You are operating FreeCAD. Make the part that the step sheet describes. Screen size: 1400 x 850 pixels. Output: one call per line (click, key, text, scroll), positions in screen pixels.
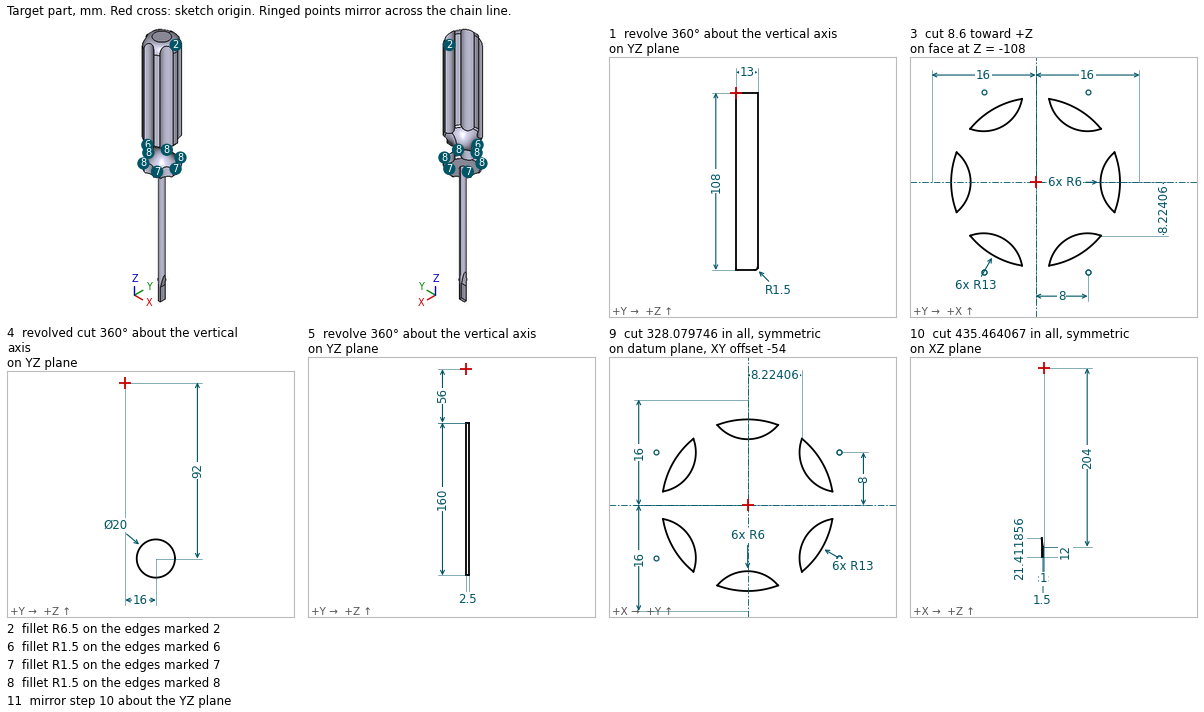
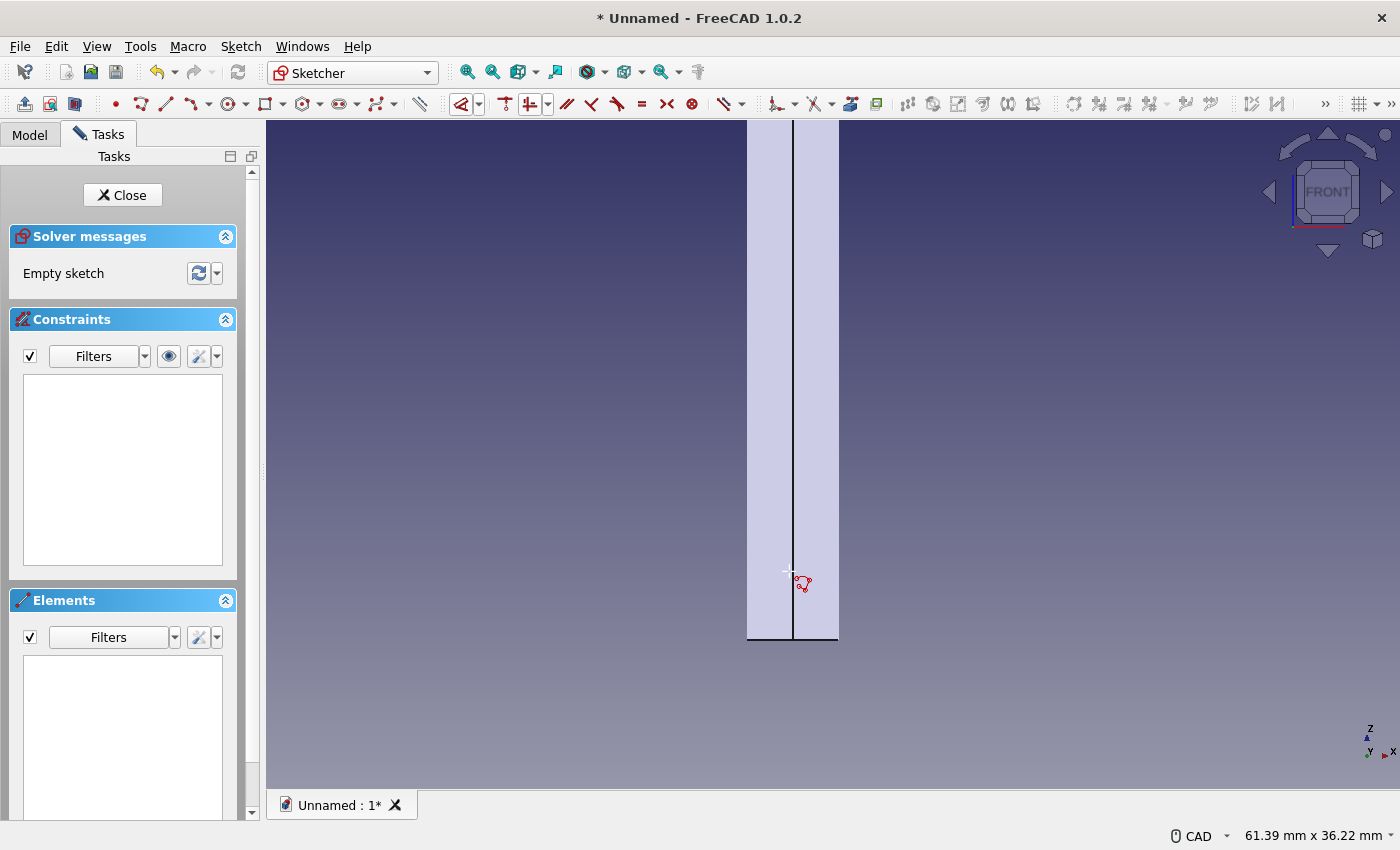
click(747, 244)
click(774, 418)
click(774, 640)
click(747, 640)
click(747, 245)
key(Escape)
key(Escape)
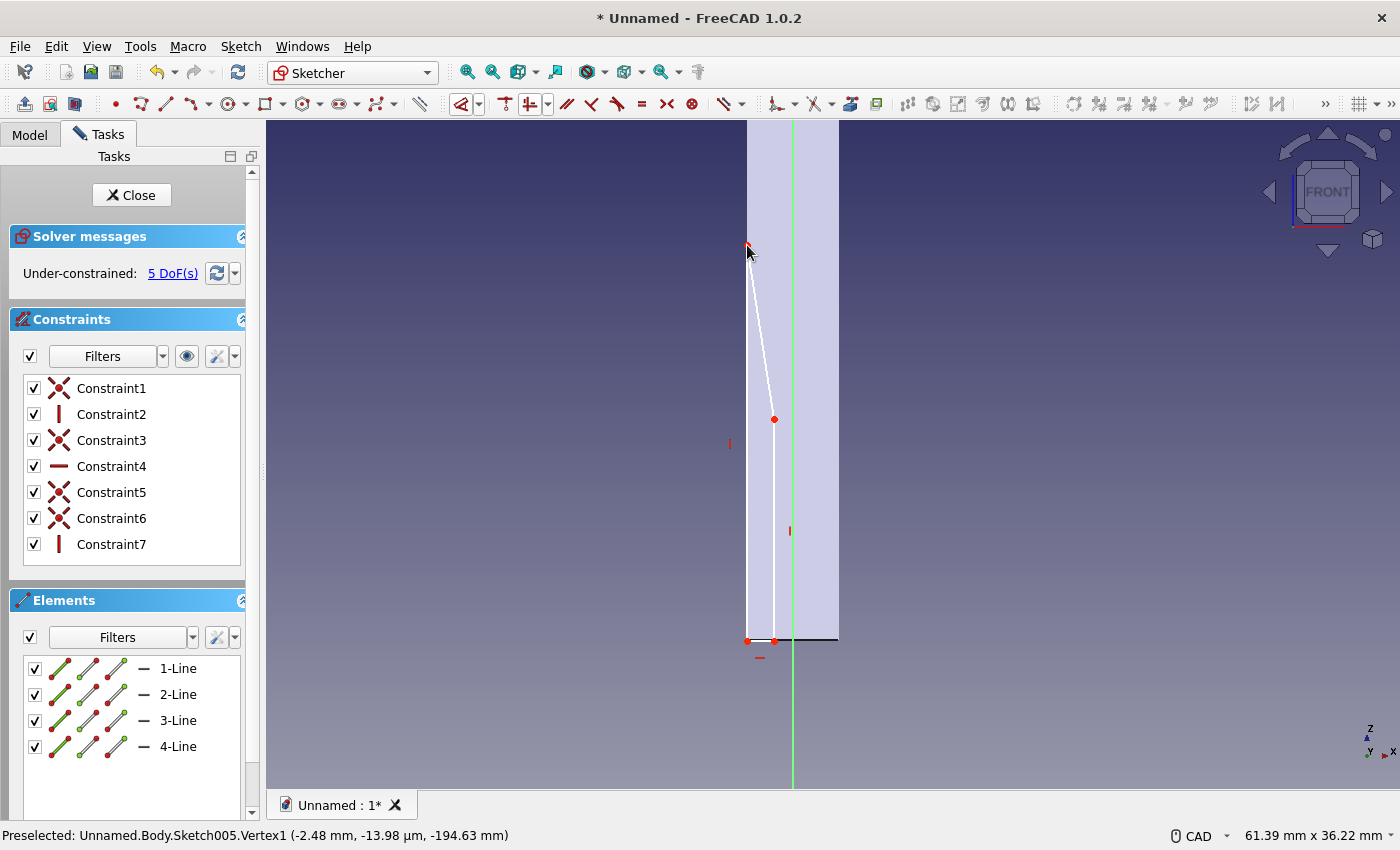
click(460, 104)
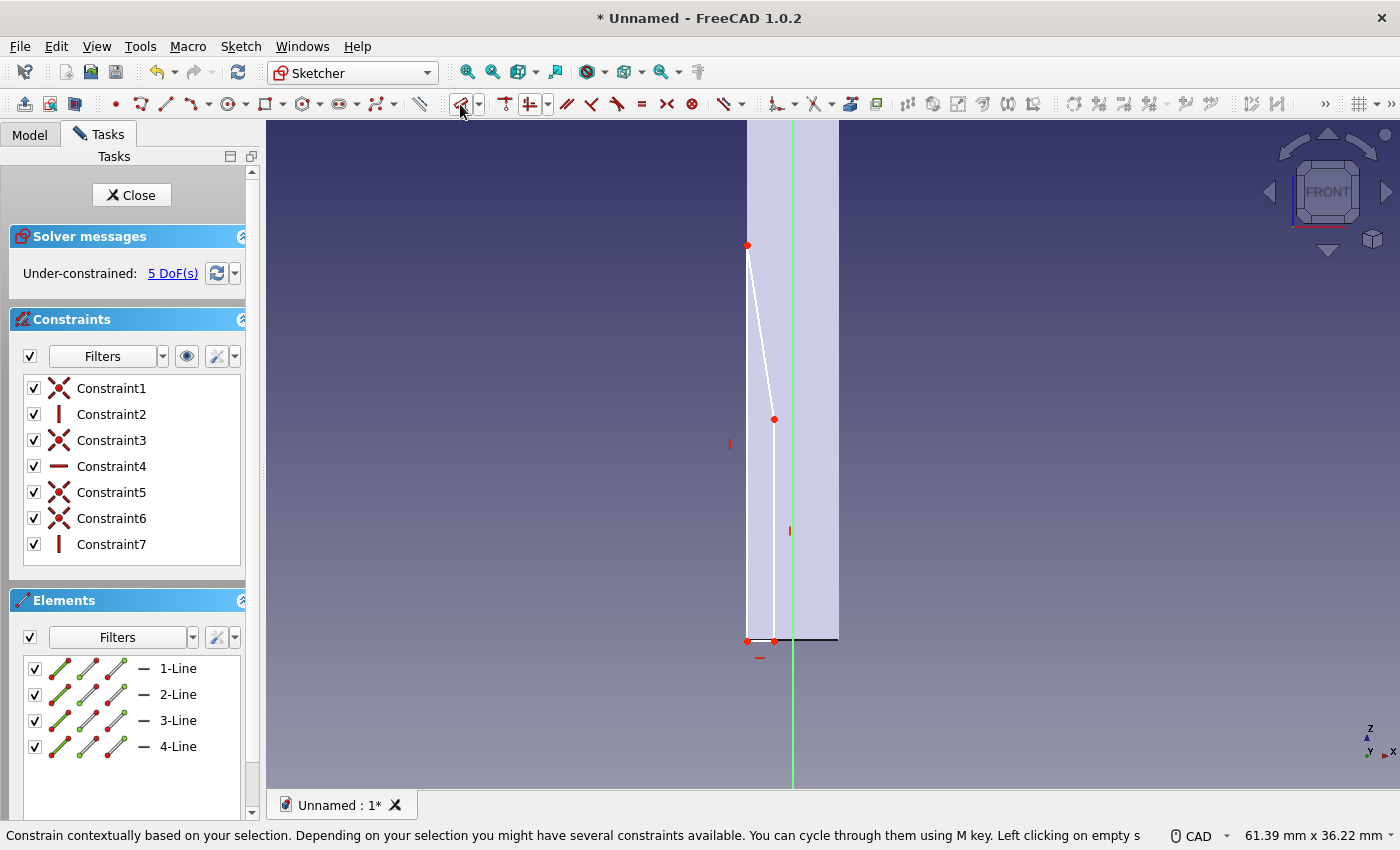
click(774, 486)
click(808, 530)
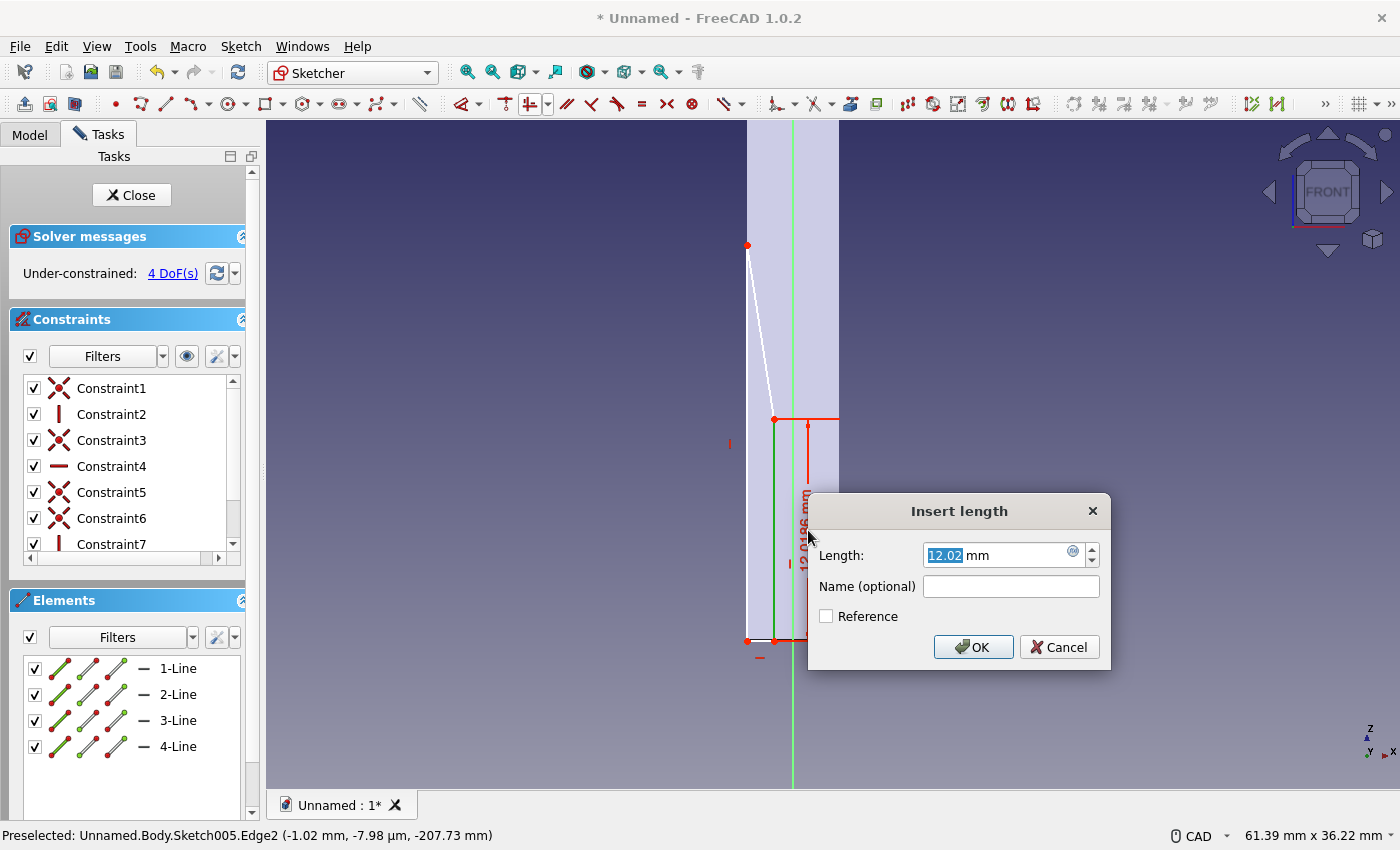
text(12)
key(Return)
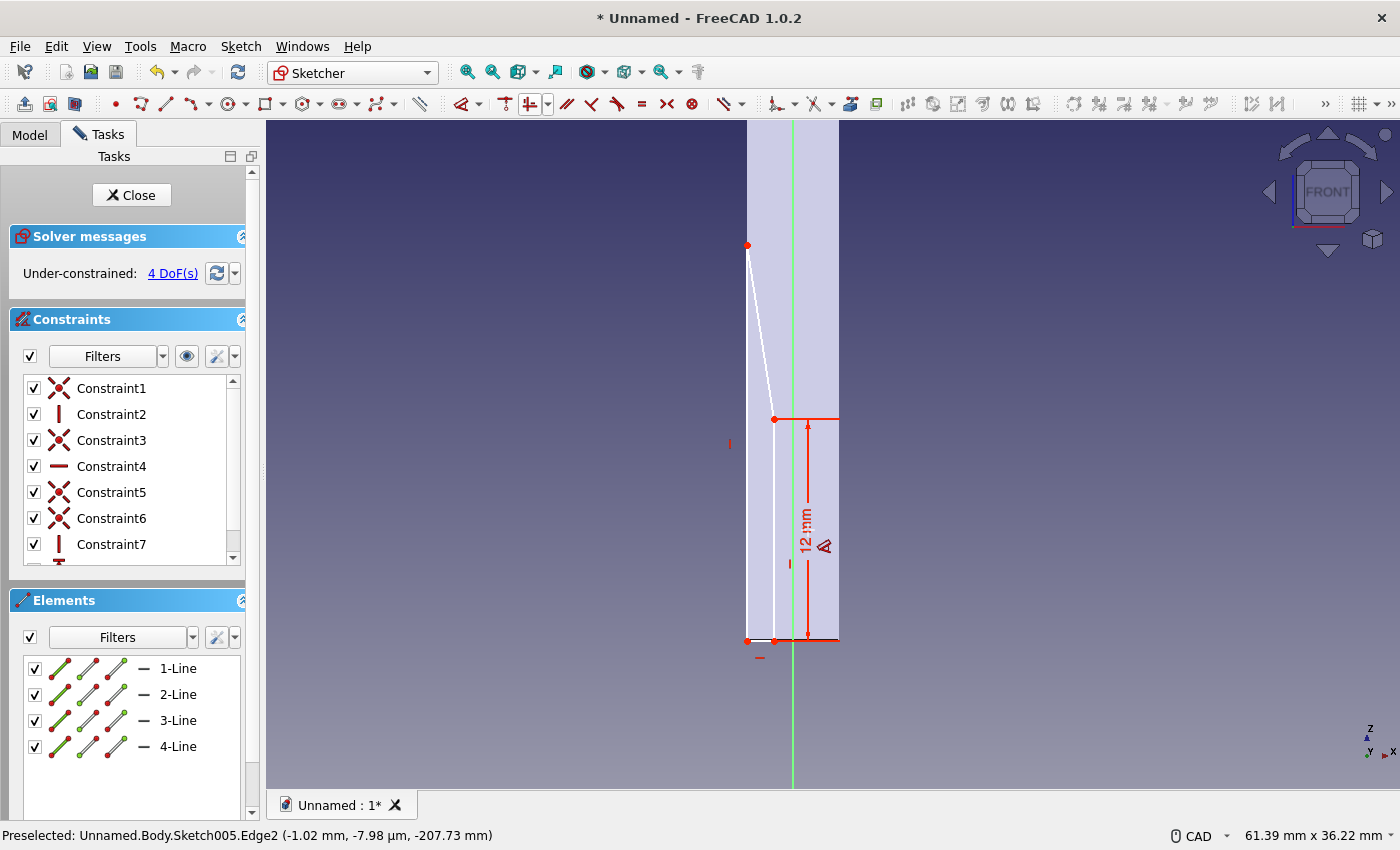
scroll(774, 419, up, 4)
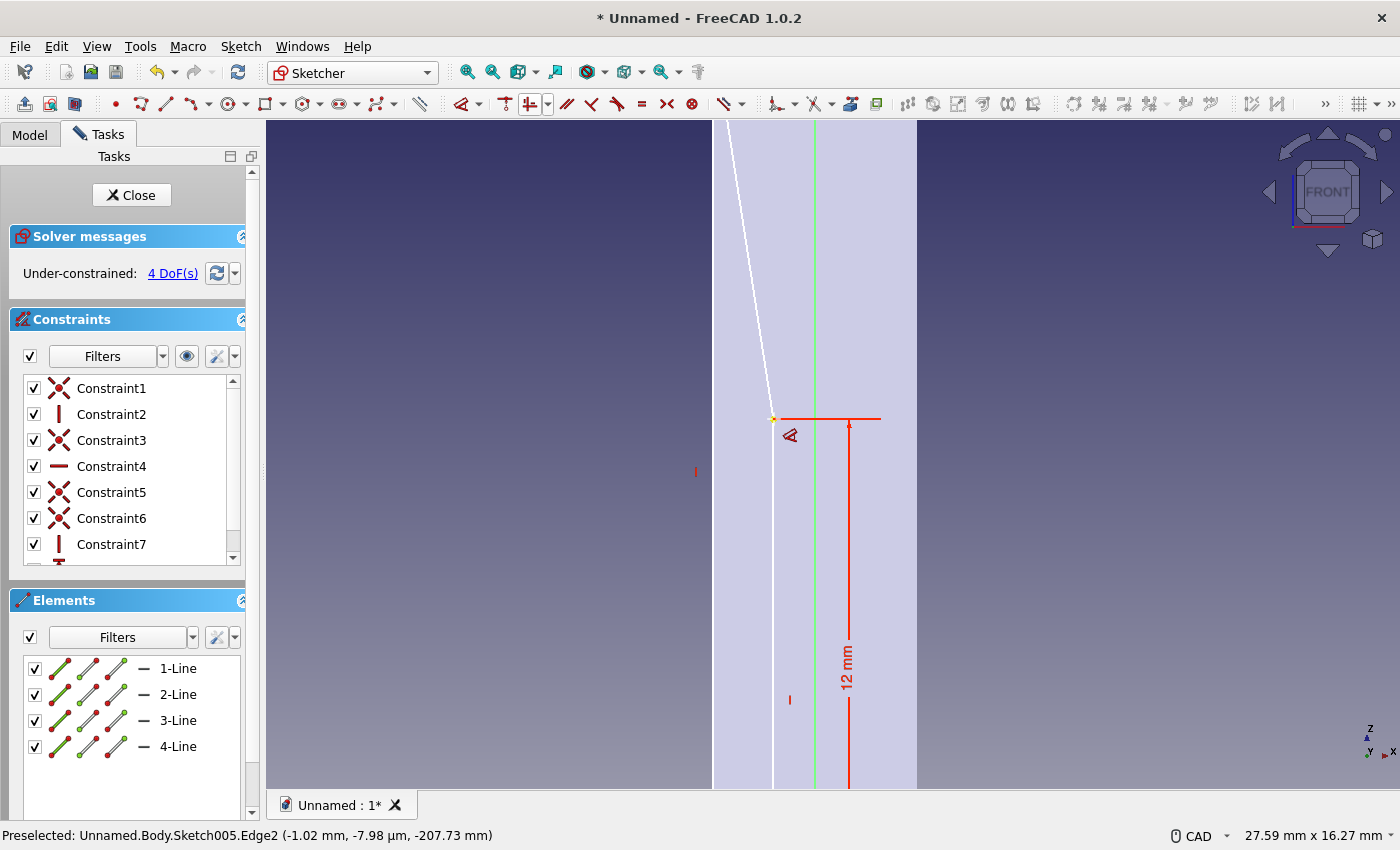
click(773, 419)
click(794, 453)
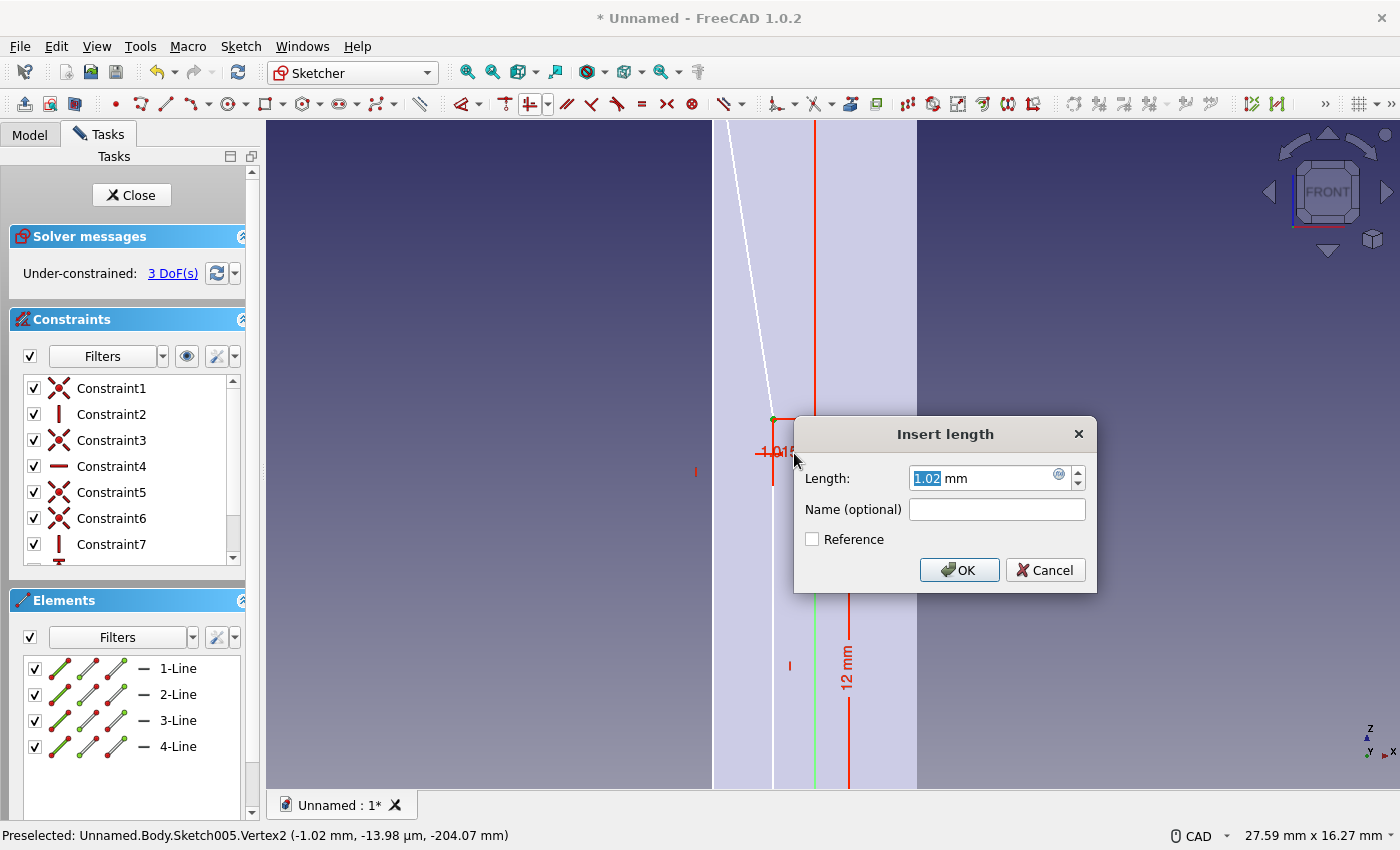
text(1)
key(Return)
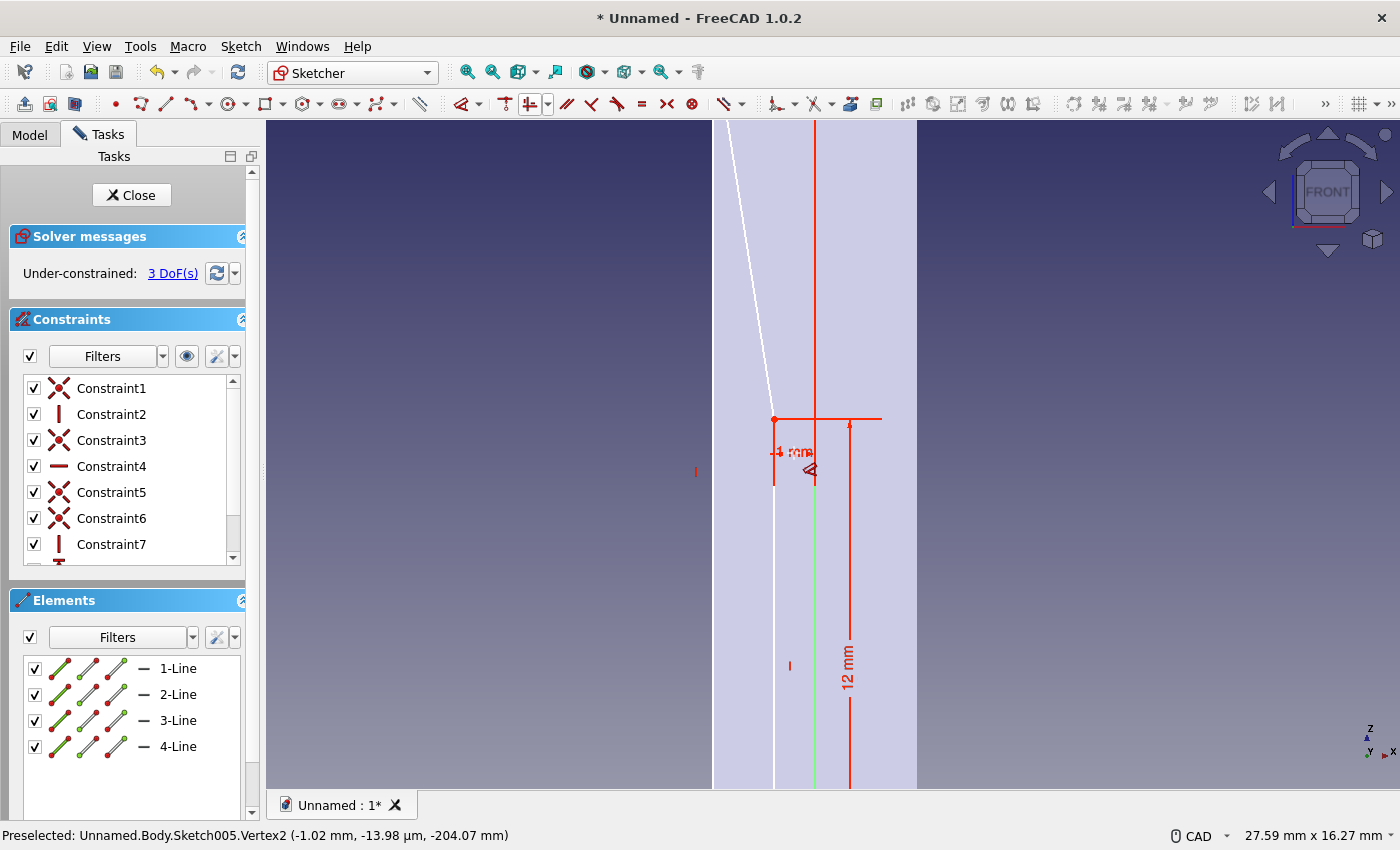
scroll(782, 442, down, 4)